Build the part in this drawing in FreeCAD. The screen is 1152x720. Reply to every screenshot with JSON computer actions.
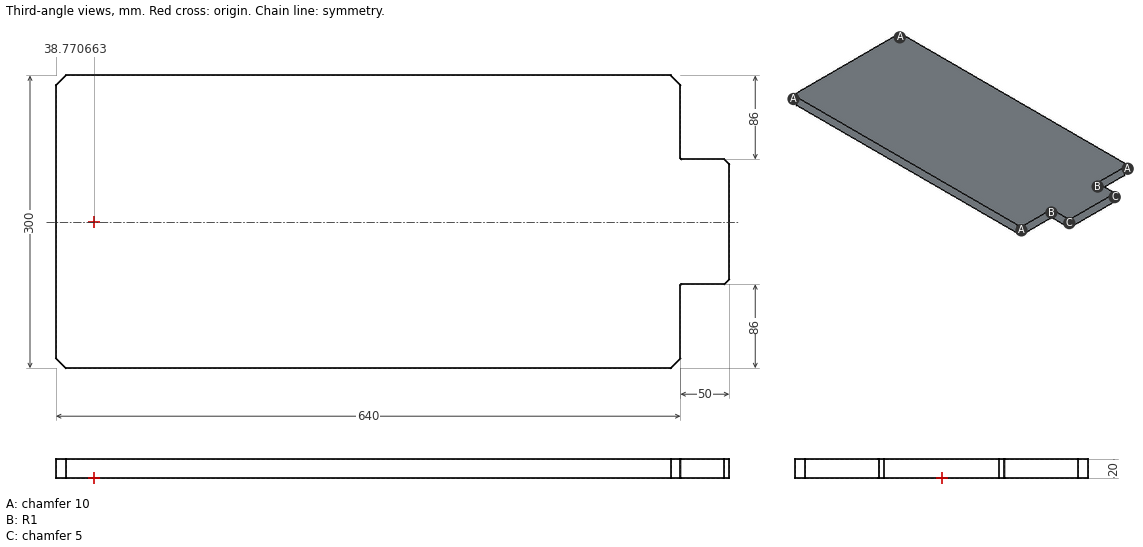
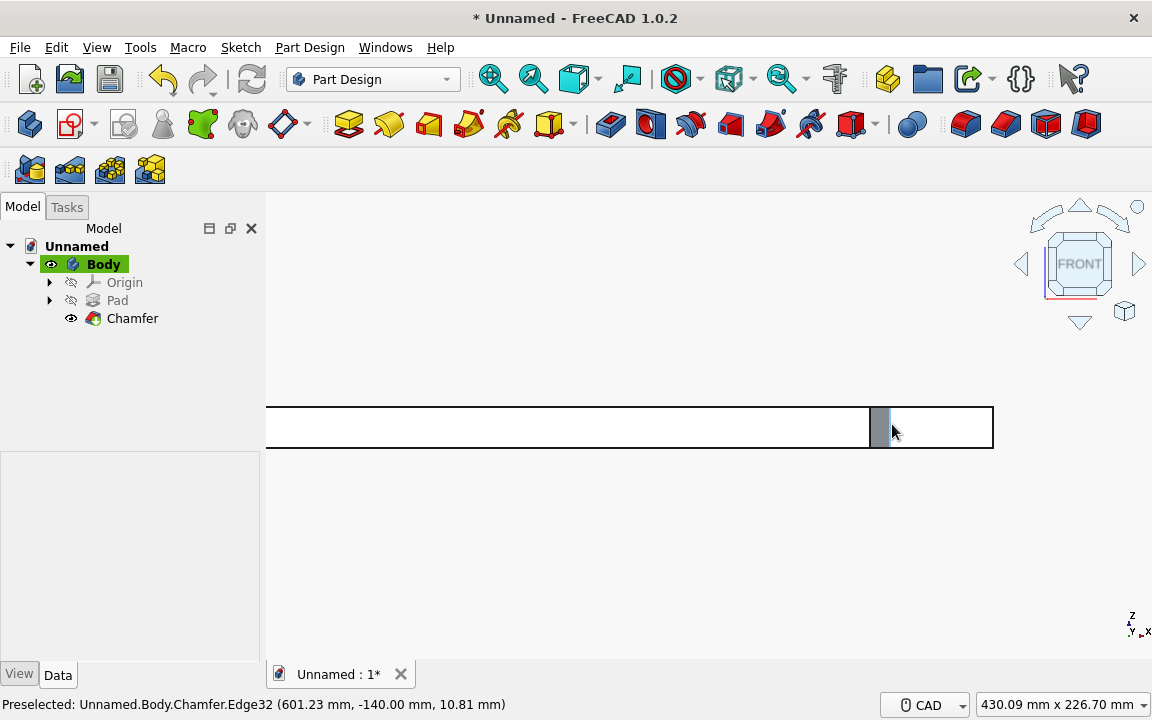
{"action": "key", "text": "v f"}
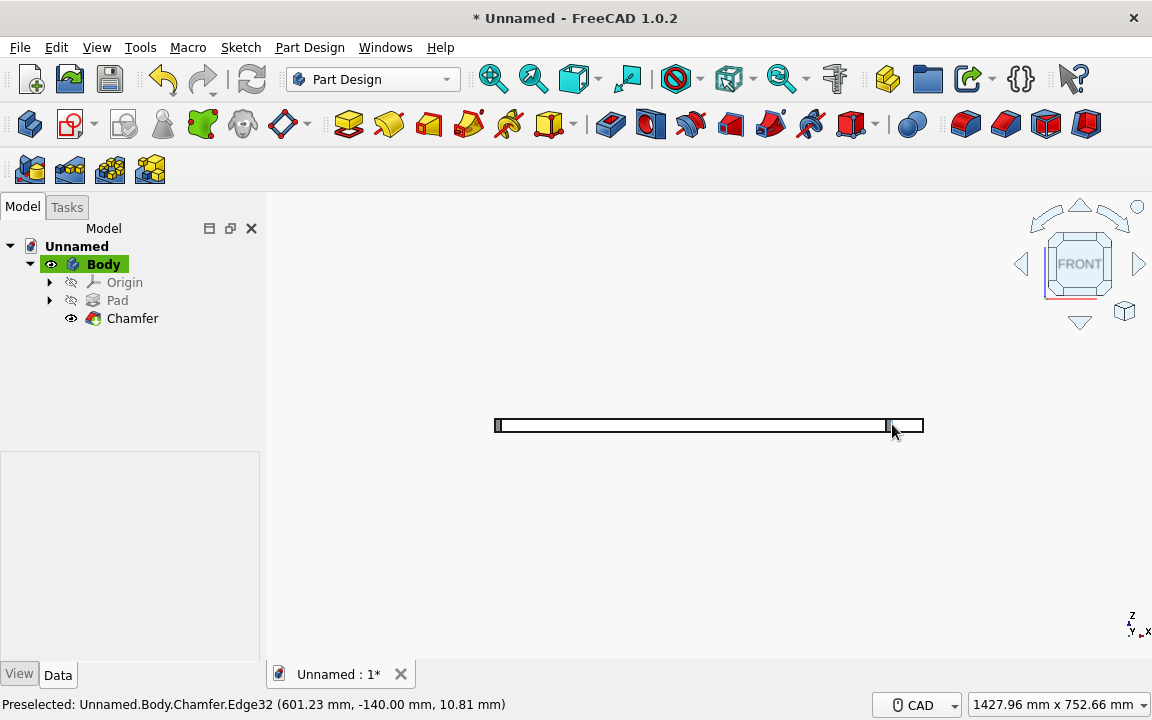
{"action": "key", "text": "3"}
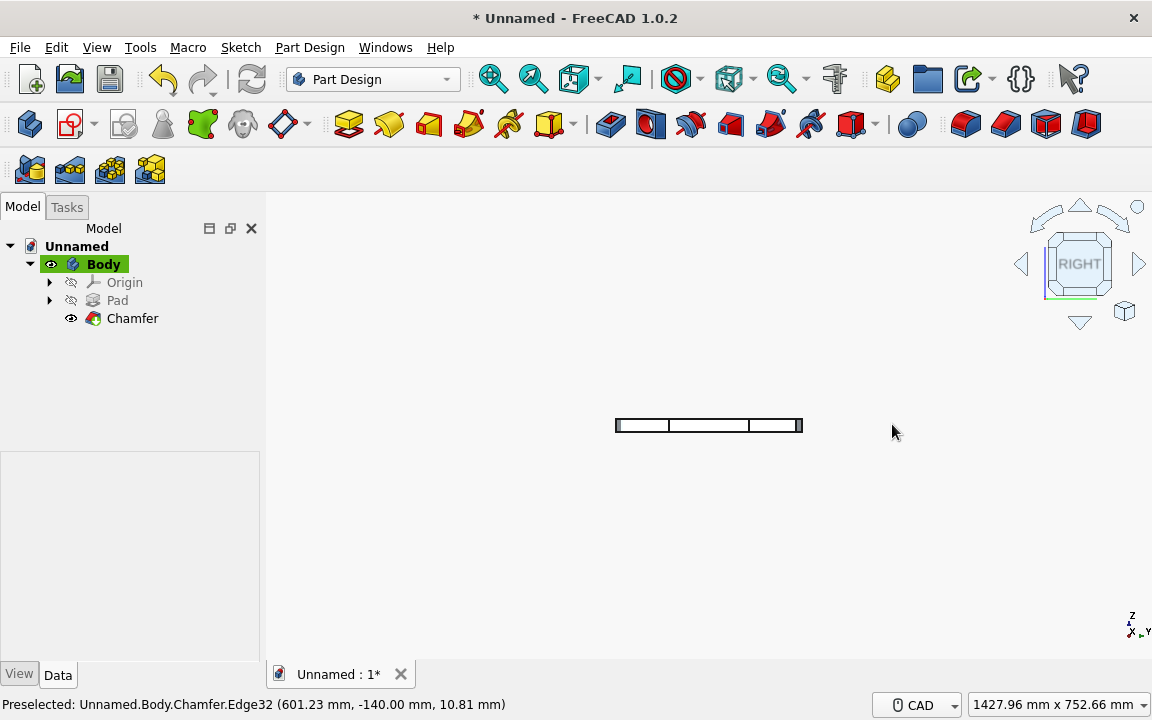
{"action": "left_click", "coordinate": [494, 80]}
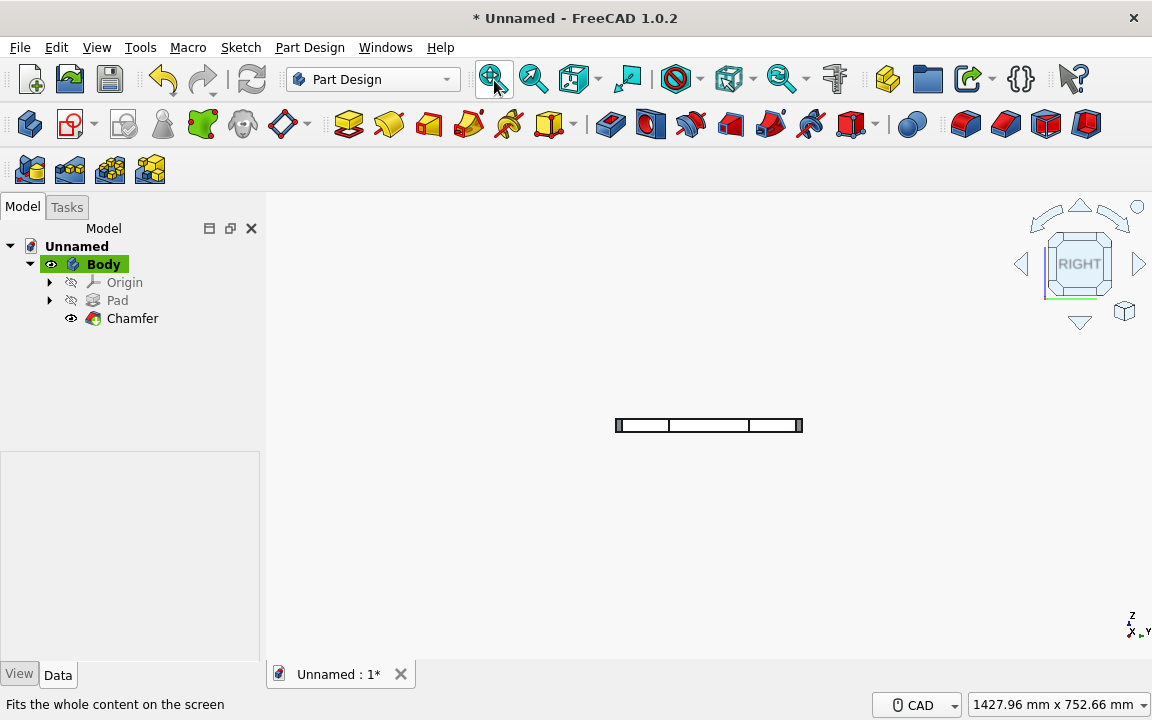
{"action": "scroll", "coordinate": [749, 424], "scroll_direction": "up", "scroll_amount": 6}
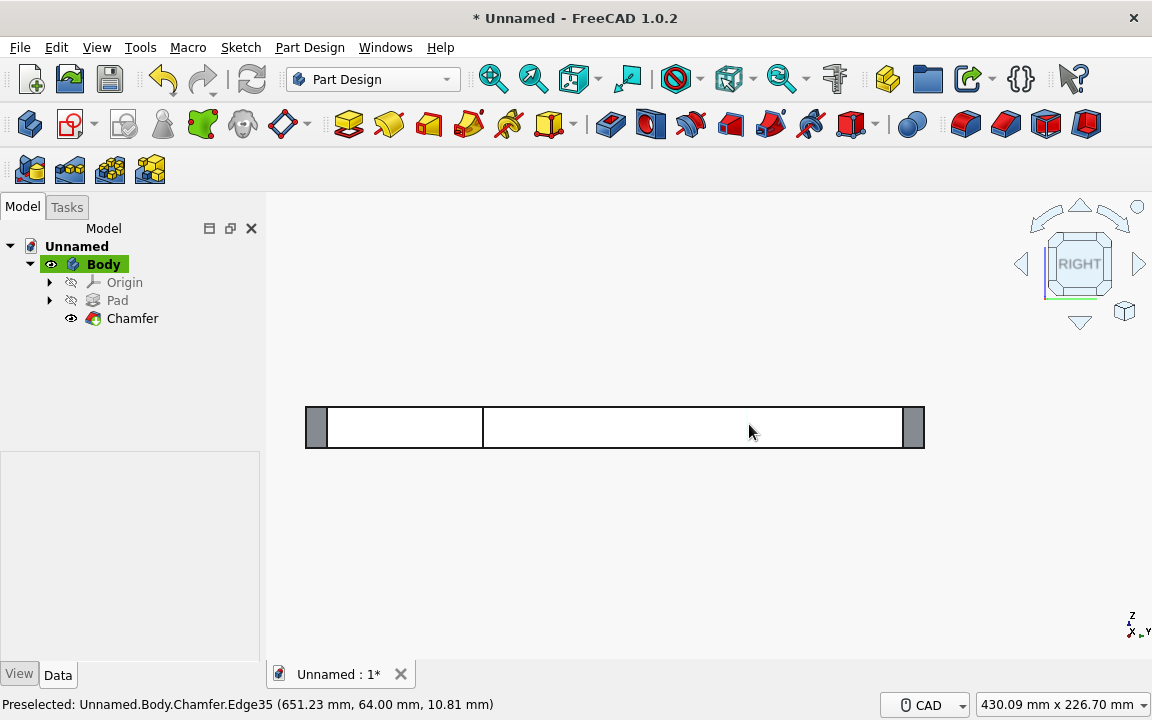
{"action": "left_click", "coordinate": [494, 80]}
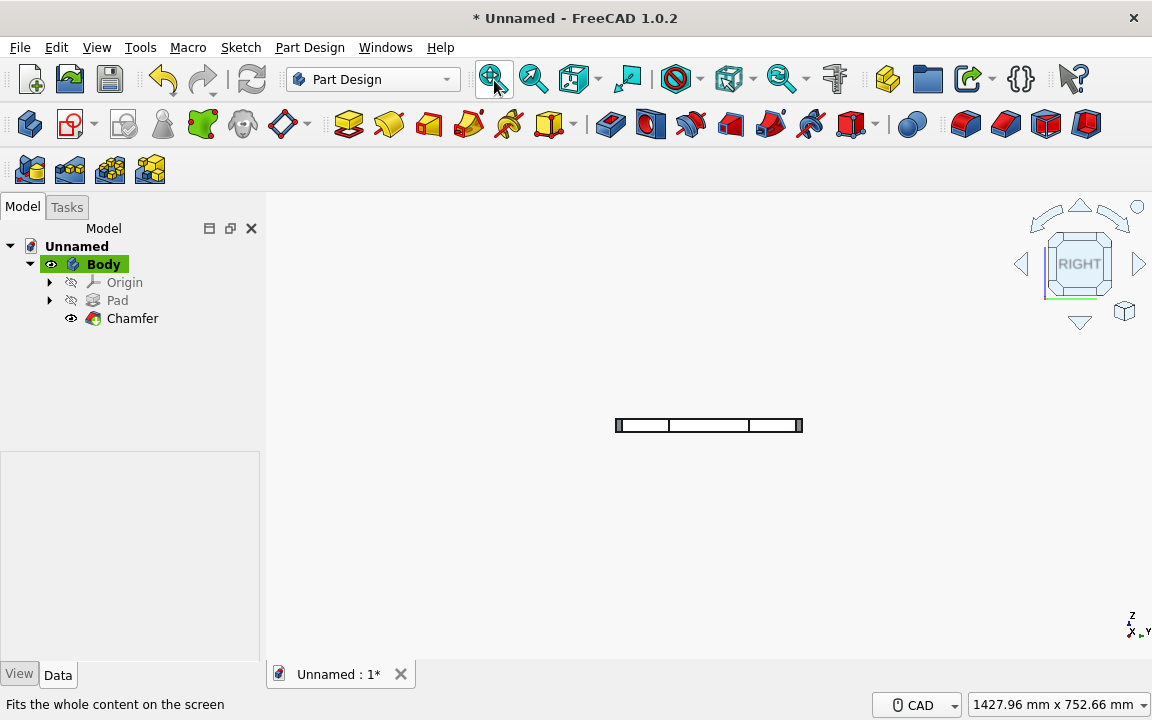
{"action": "key", "text": "5"}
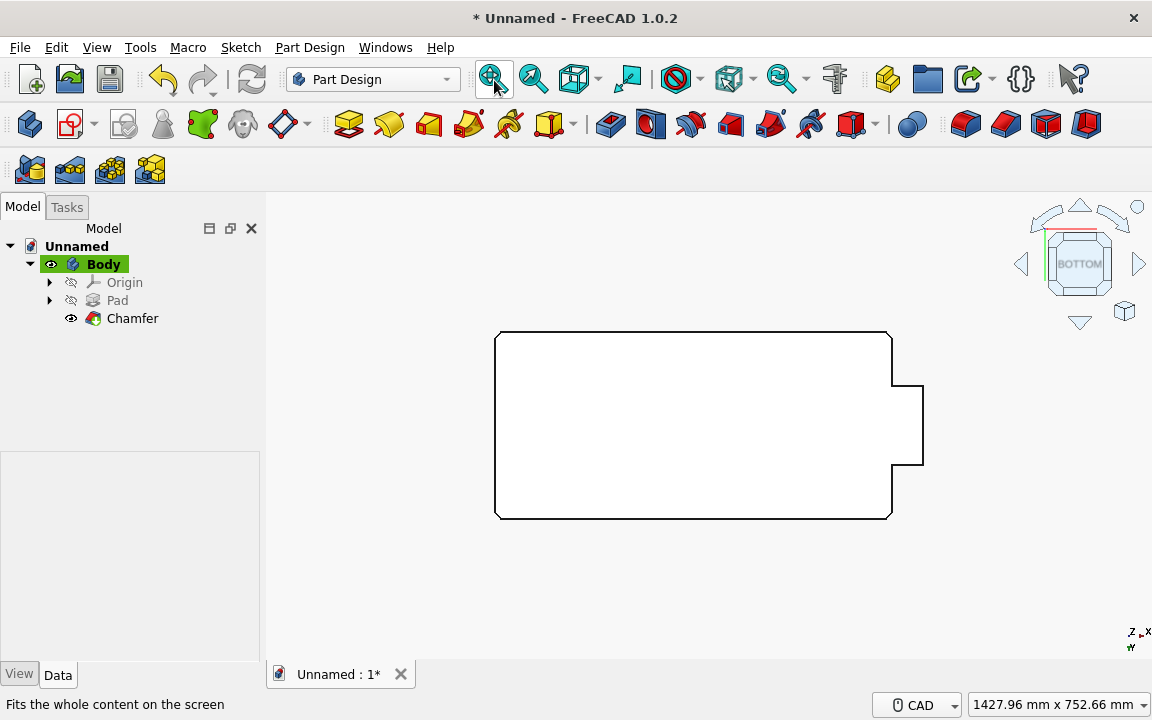
{"action": "scroll", "coordinate": [892, 464], "scroll_direction": "up", "scroll_amount": 6}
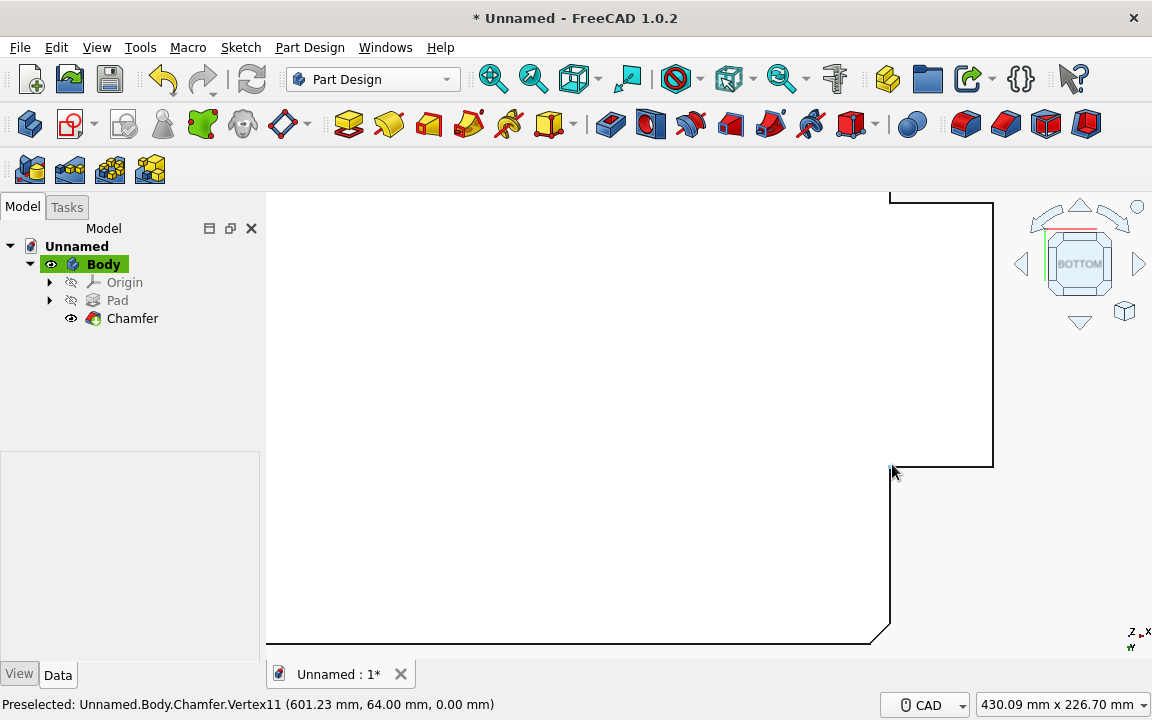
{"action": "key", "text": "v f"}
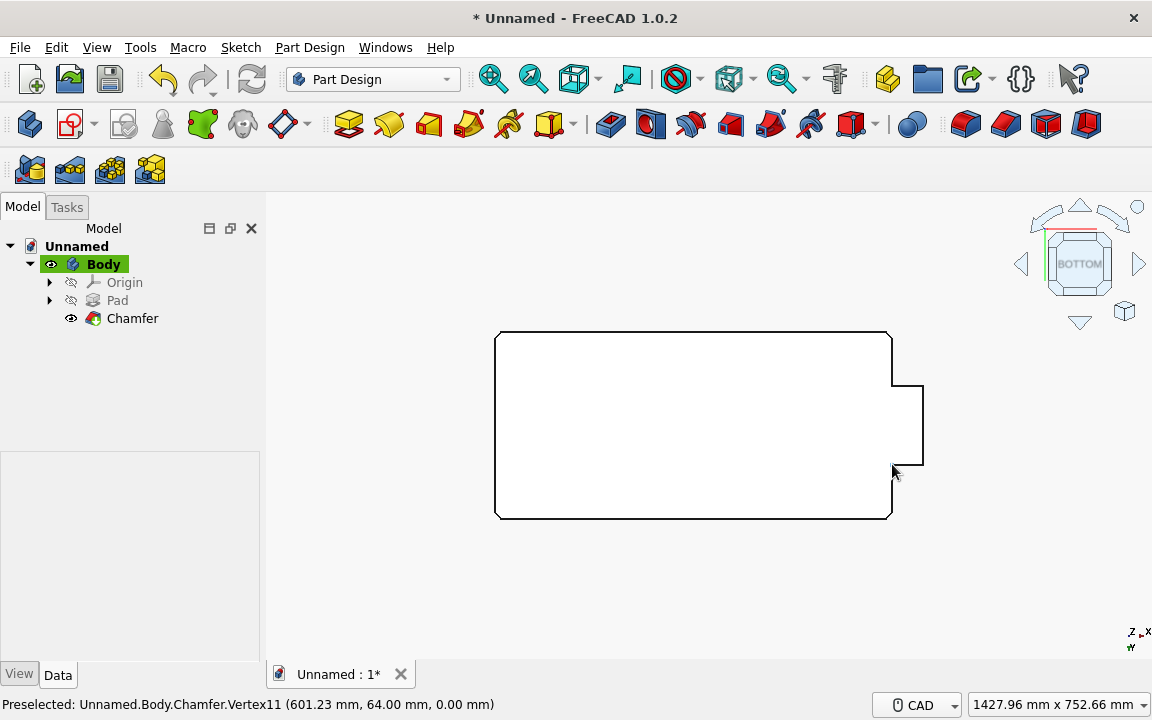
{"action": "key", "text": "4"}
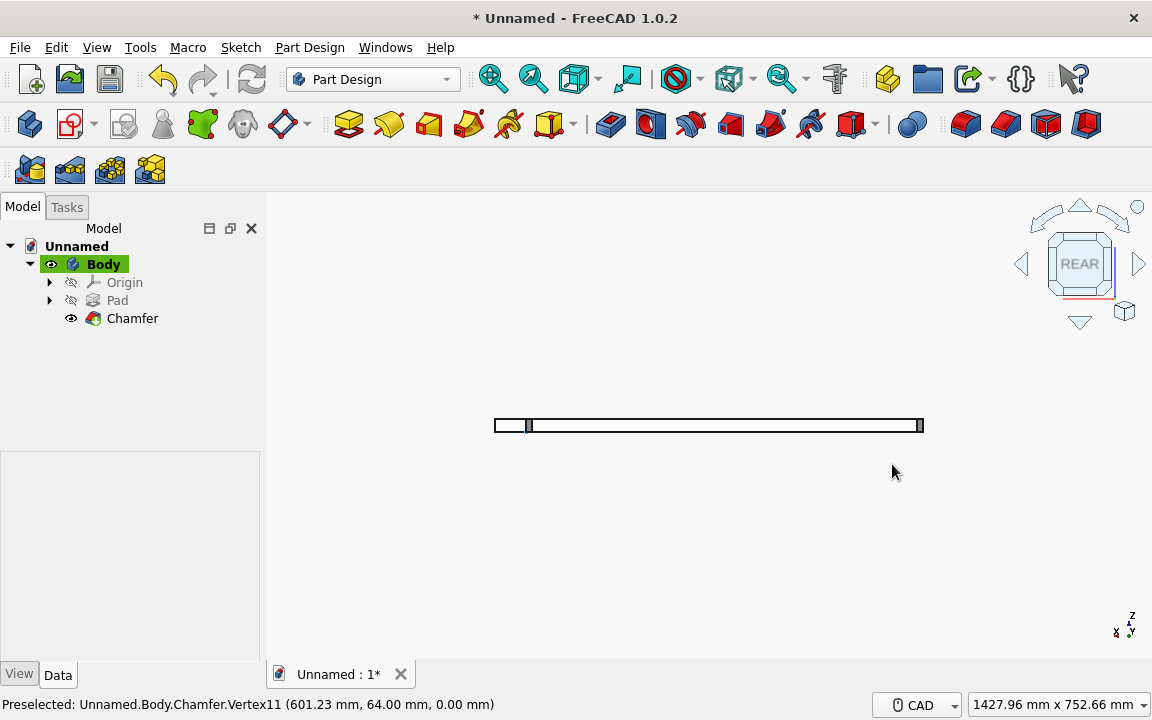
{"action": "scroll", "coordinate": [526, 424], "scroll_direction": "up", "scroll_amount": 6}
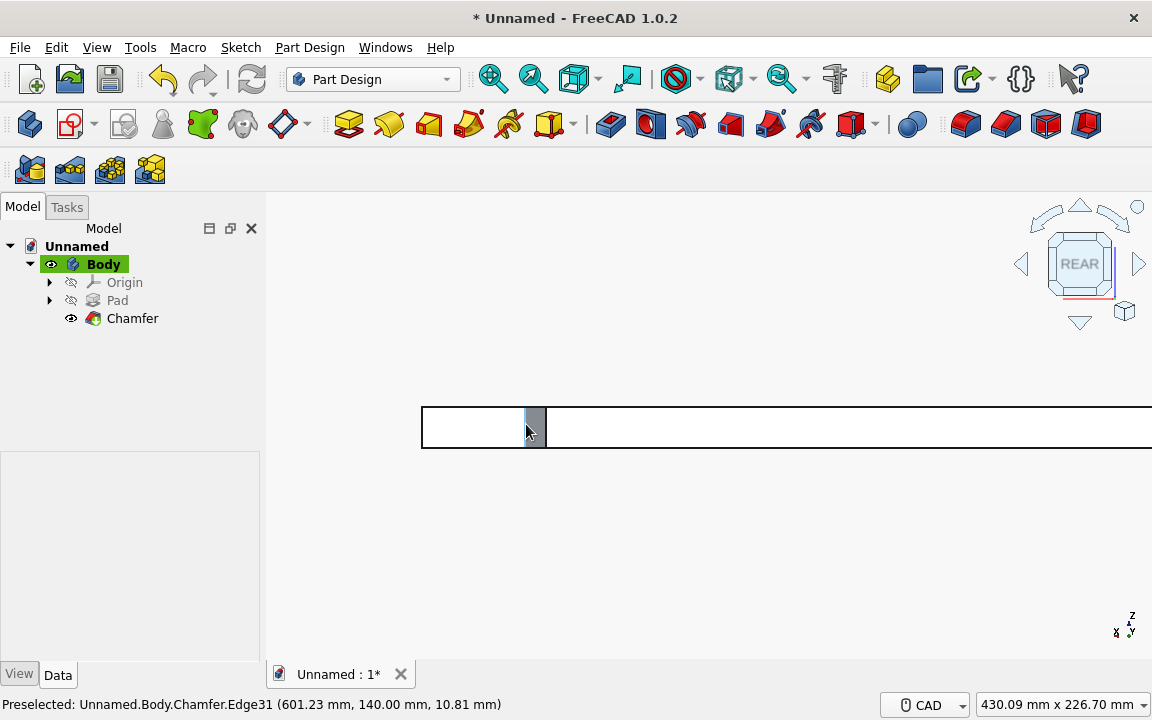
{"action": "left_click", "coordinate": [494, 80]}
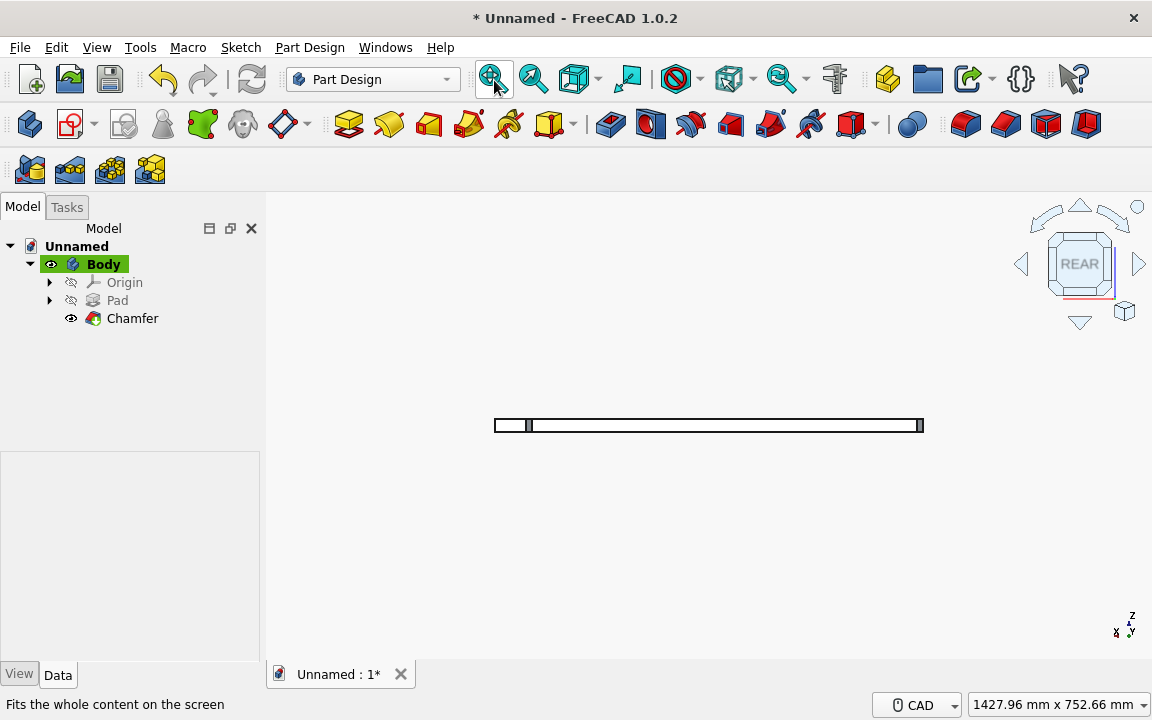
{"action": "key", "text": "6"}